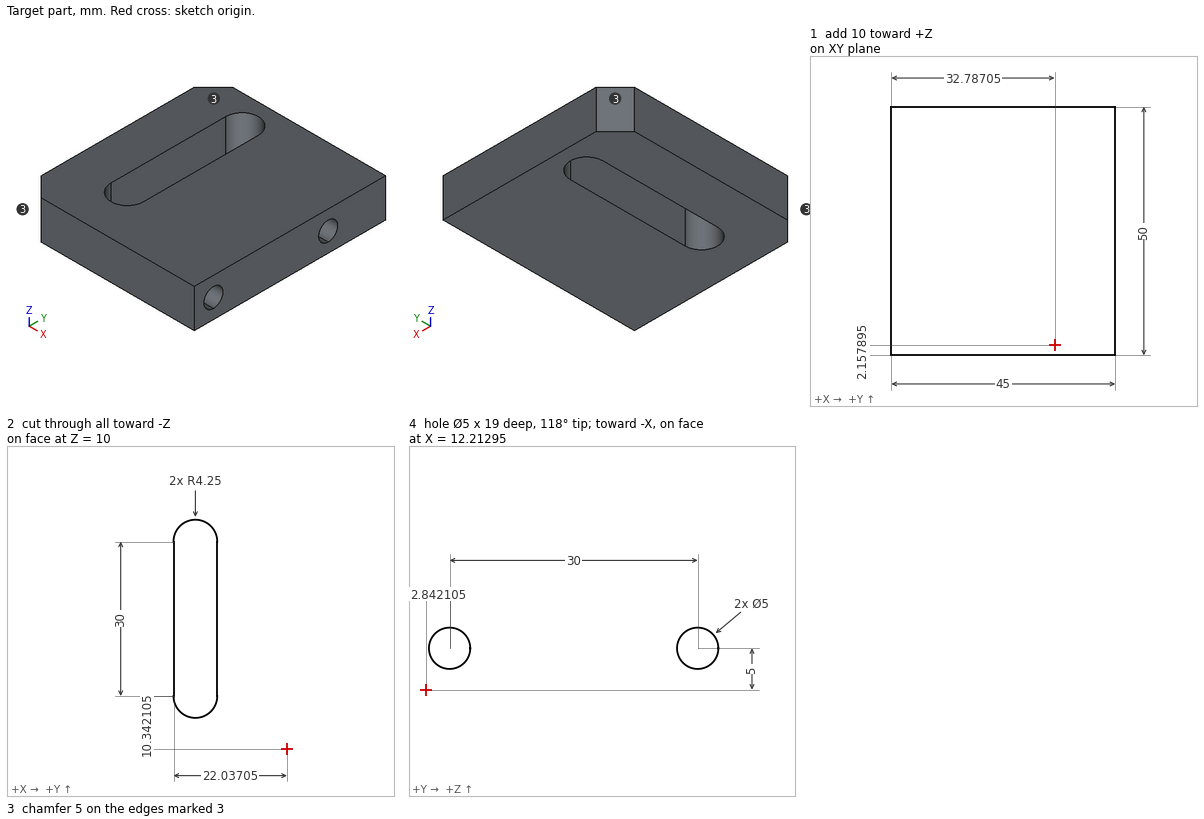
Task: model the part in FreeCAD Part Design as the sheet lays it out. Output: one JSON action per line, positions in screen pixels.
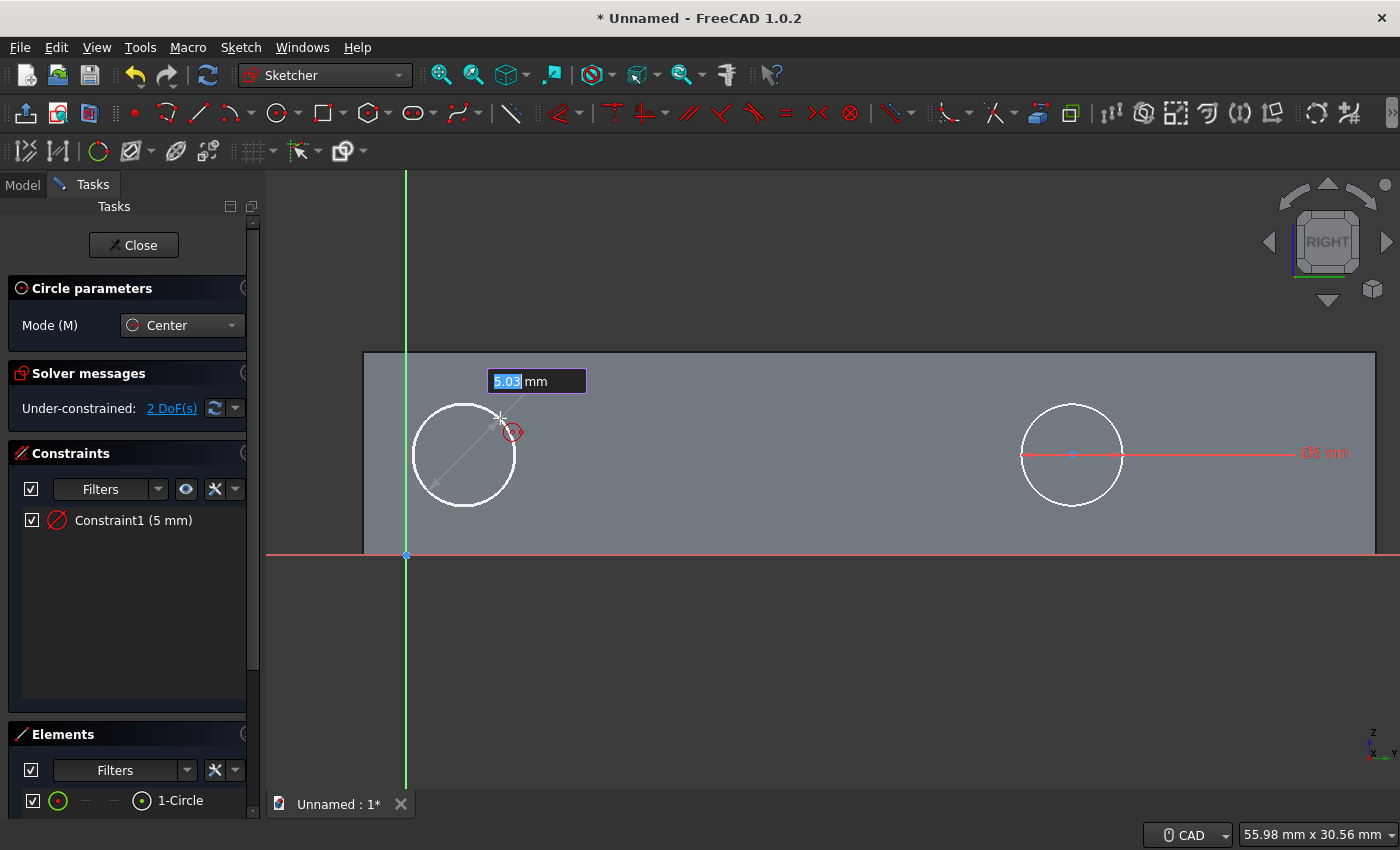
{"action": "type", "text": "5"}
{"action": "key", "text": "Return"}
{"action": "key", "text": "Escape"}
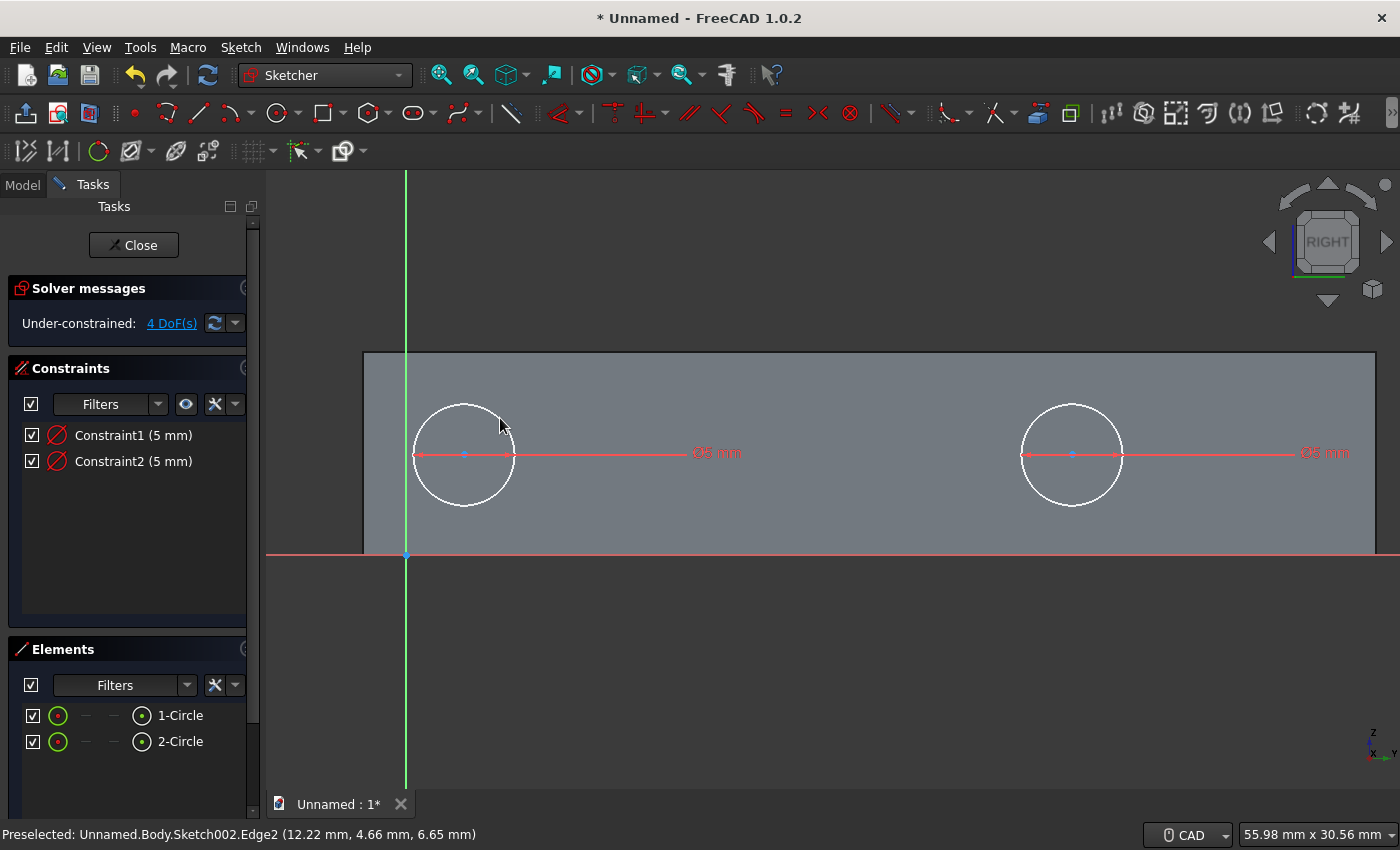
{"action": "left_click", "coordinate": [1072, 455]}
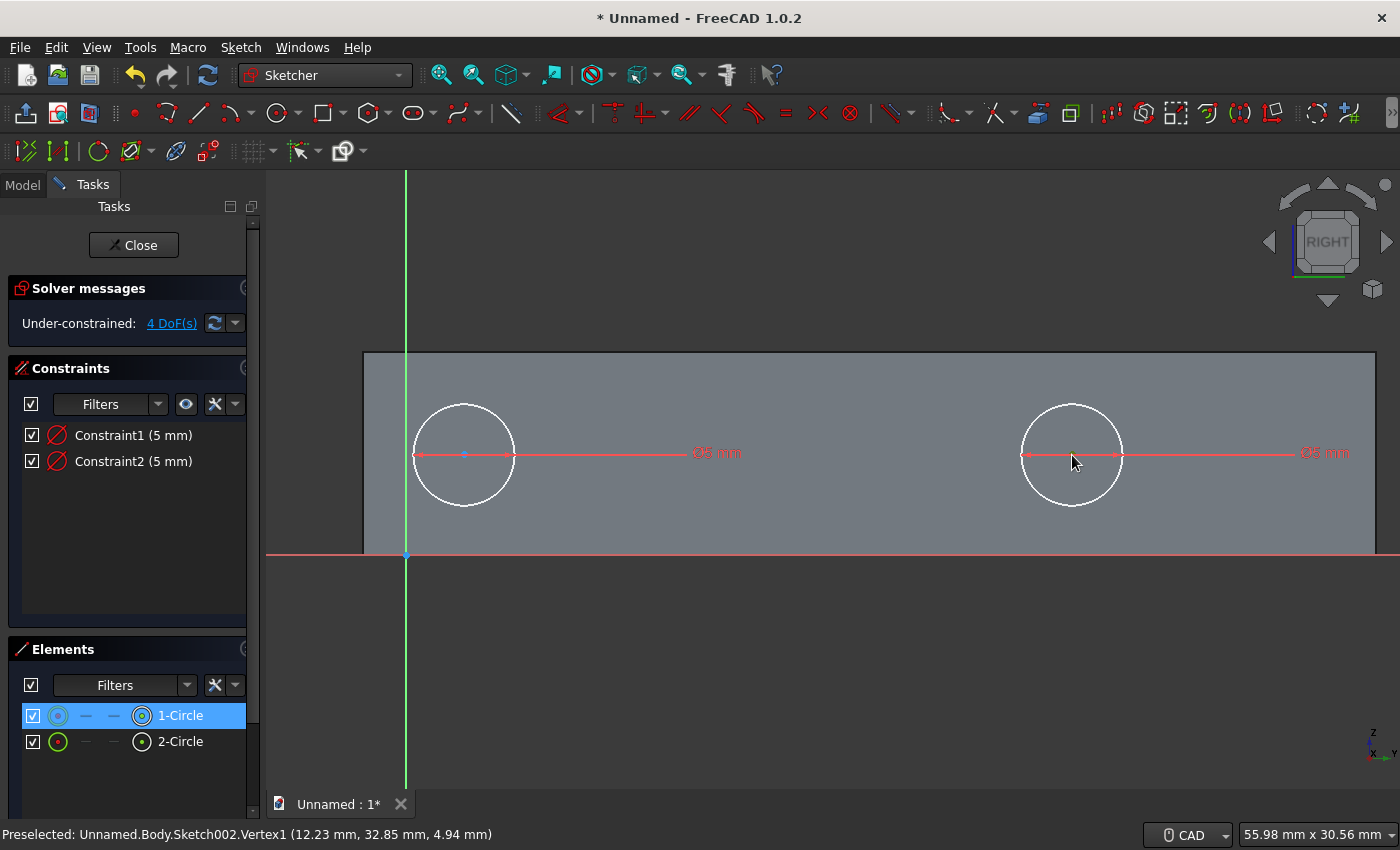
{"action": "left_click", "coordinate": [464, 455]}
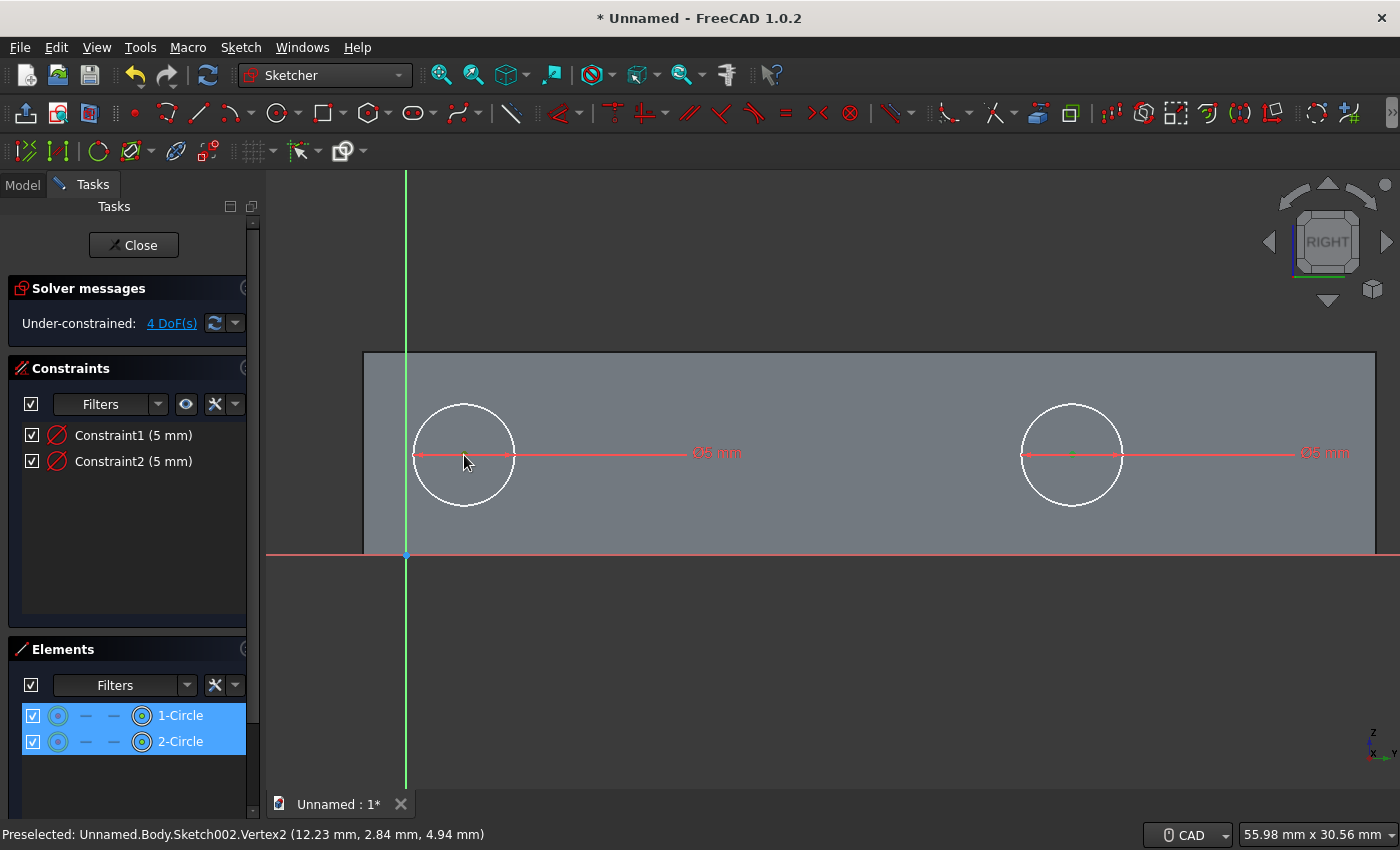
{"action": "left_click", "coordinate": [668, 114]}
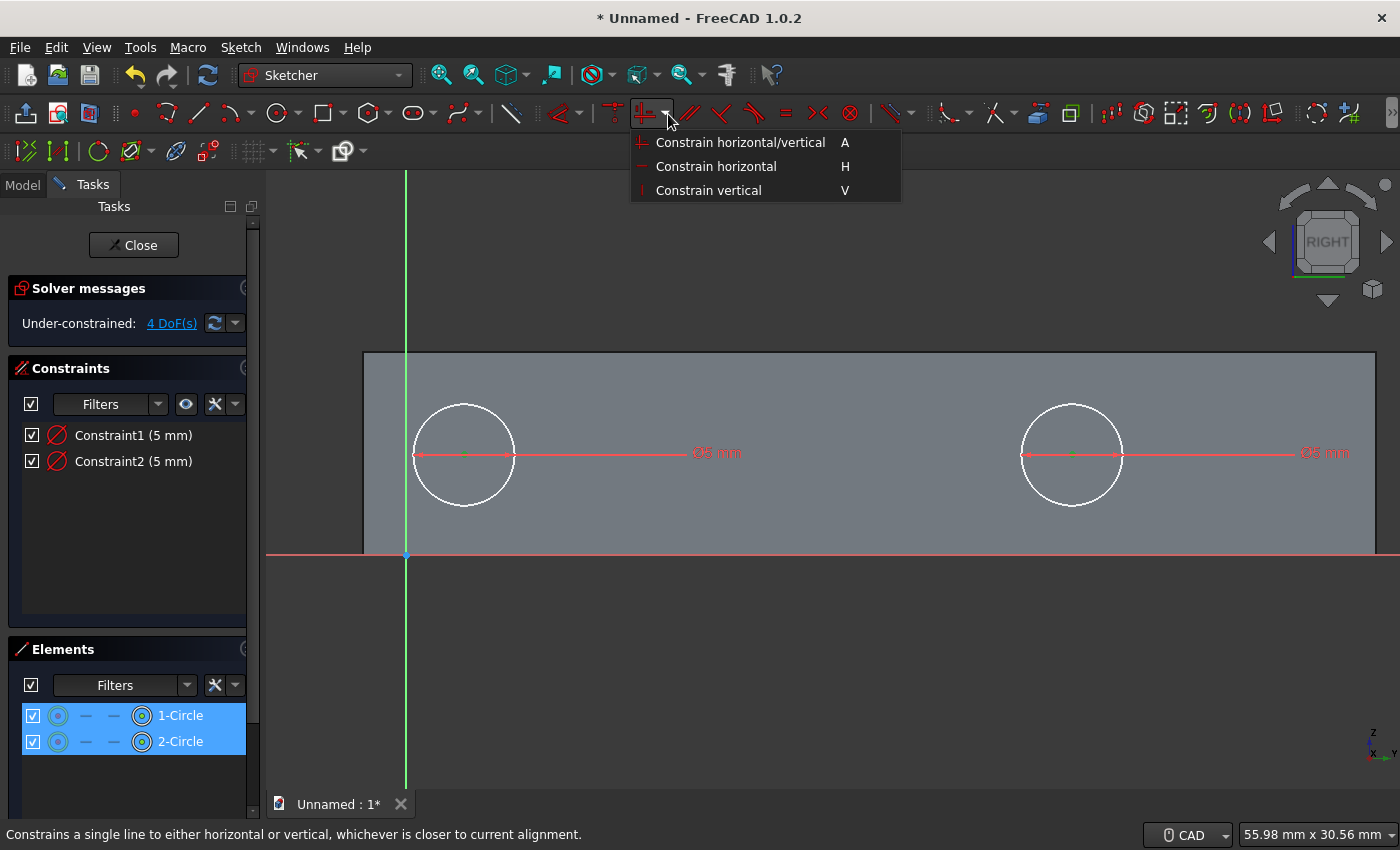
{"action": "left_click", "coordinate": [766, 166]}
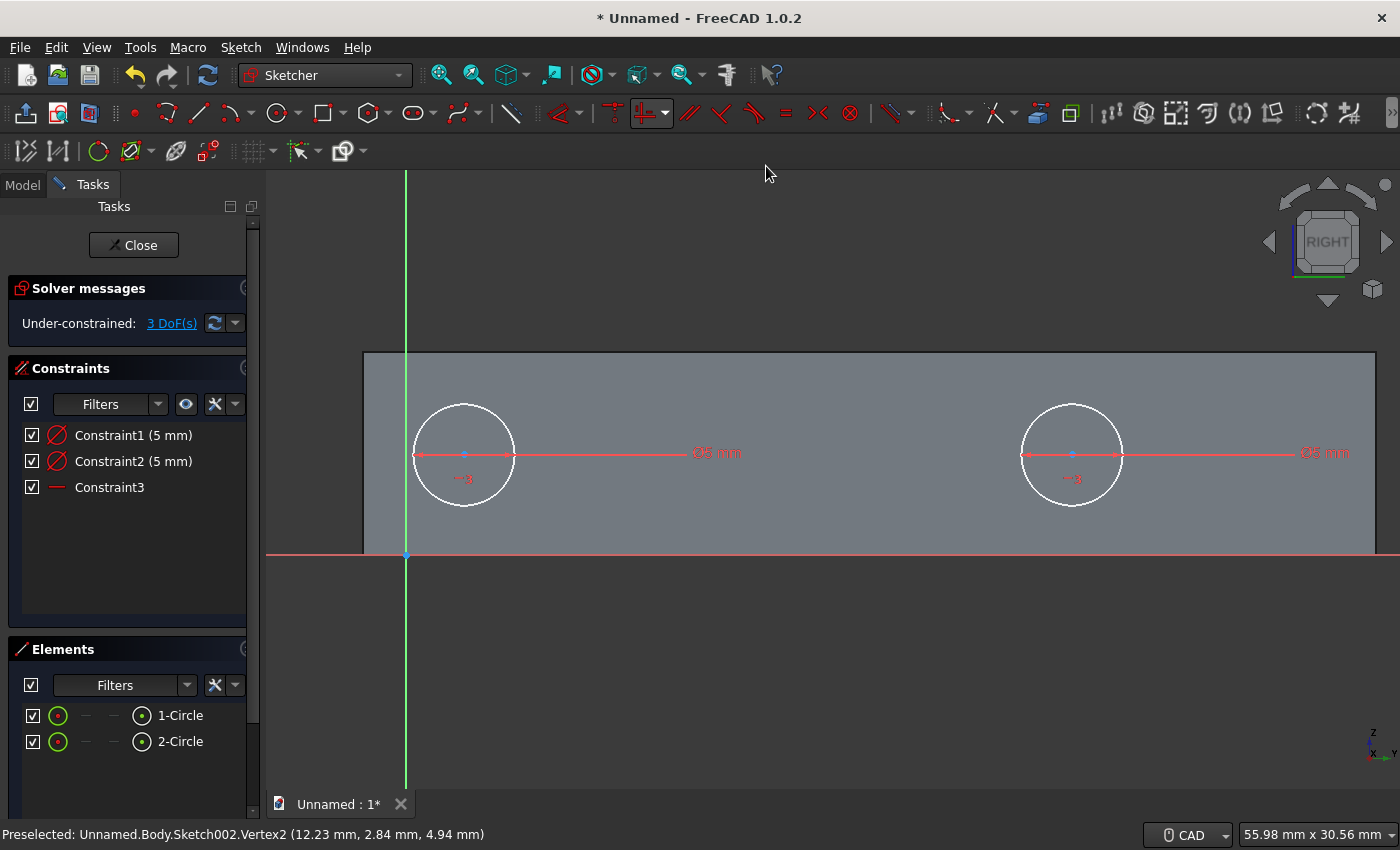
{"action": "left_click", "coordinate": [558, 114]}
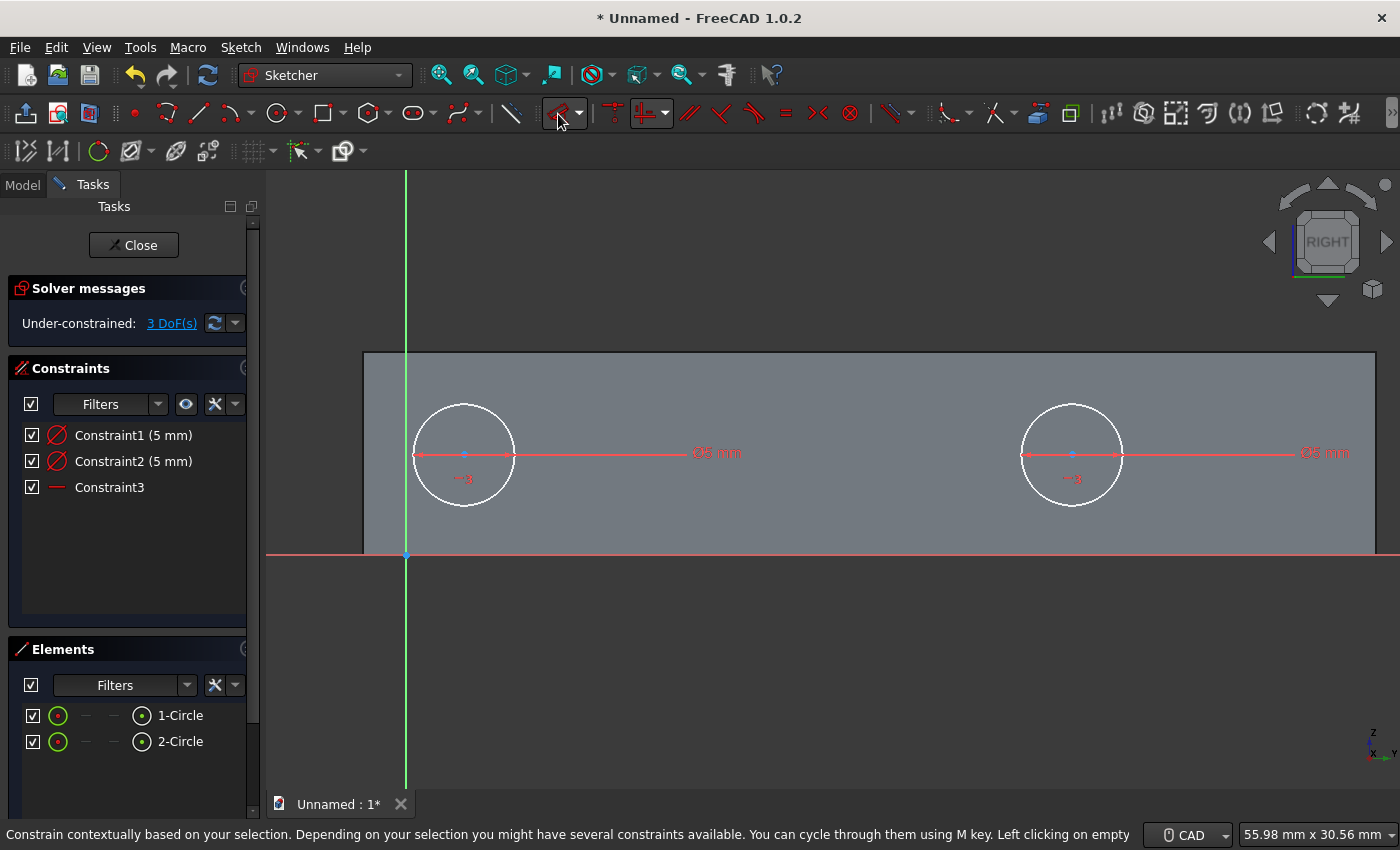
{"action": "left_click", "coordinate": [1072, 455]}
{"action": "left_click", "coordinate": [372, 505]}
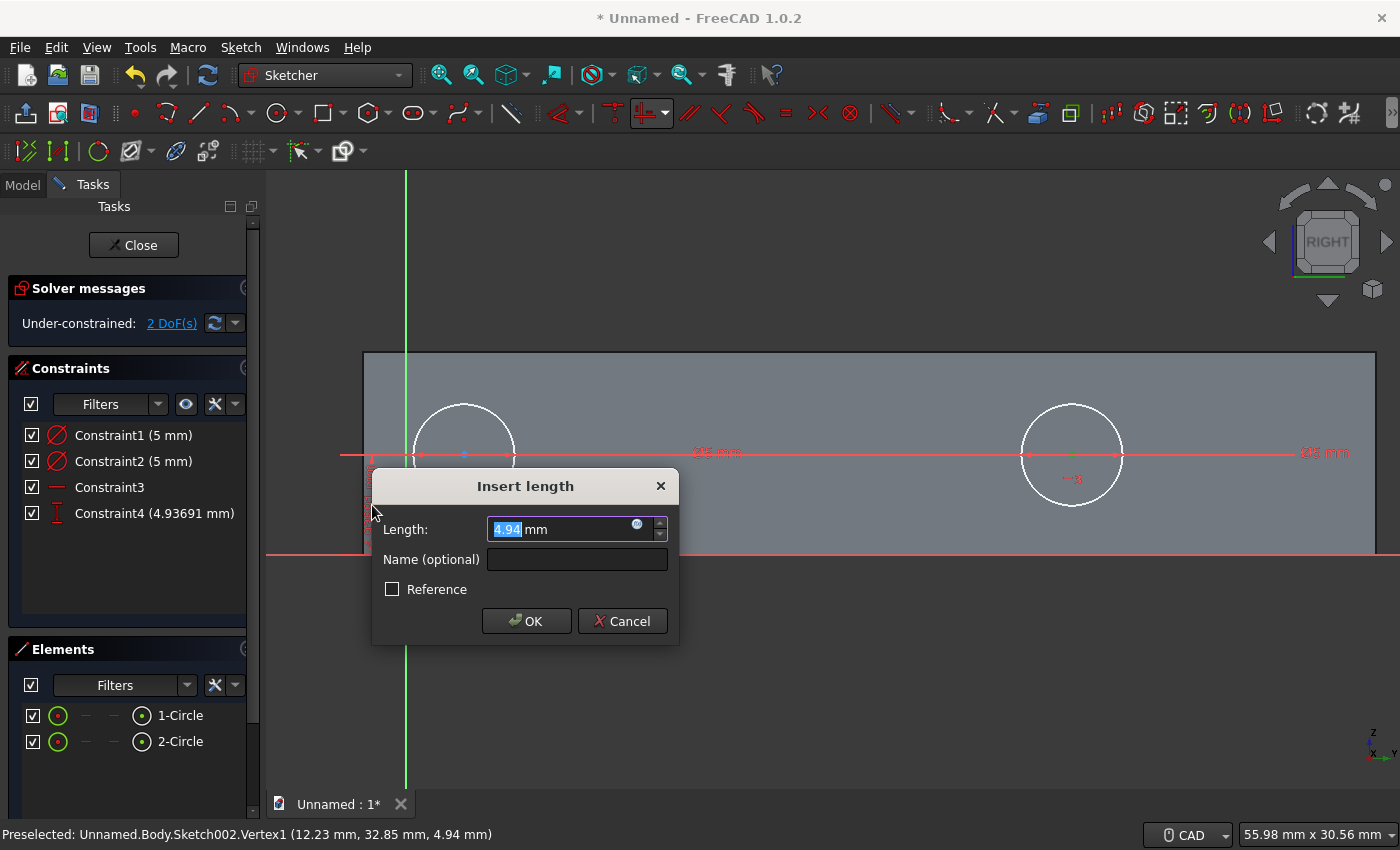
{"action": "type", "text": "5"}
{"action": "key", "text": "Return"}